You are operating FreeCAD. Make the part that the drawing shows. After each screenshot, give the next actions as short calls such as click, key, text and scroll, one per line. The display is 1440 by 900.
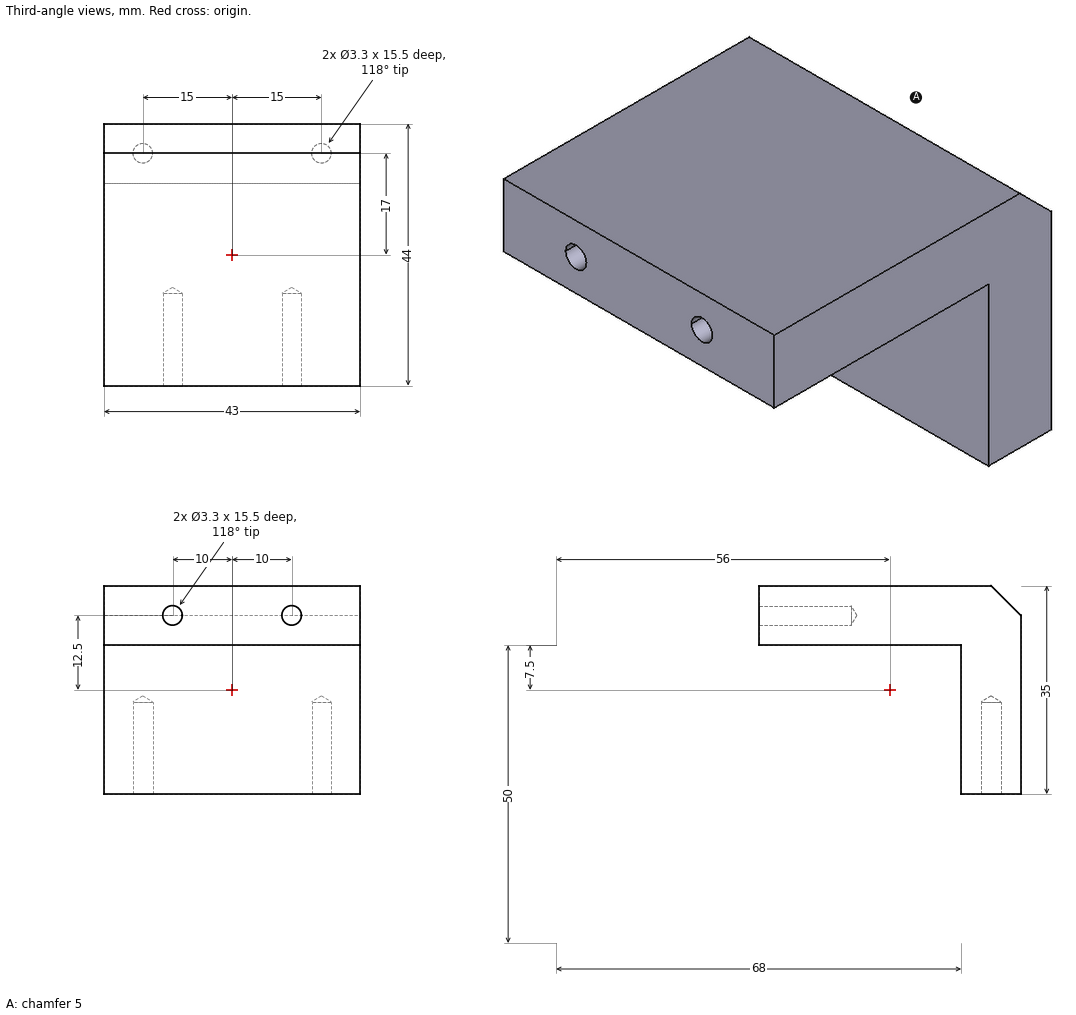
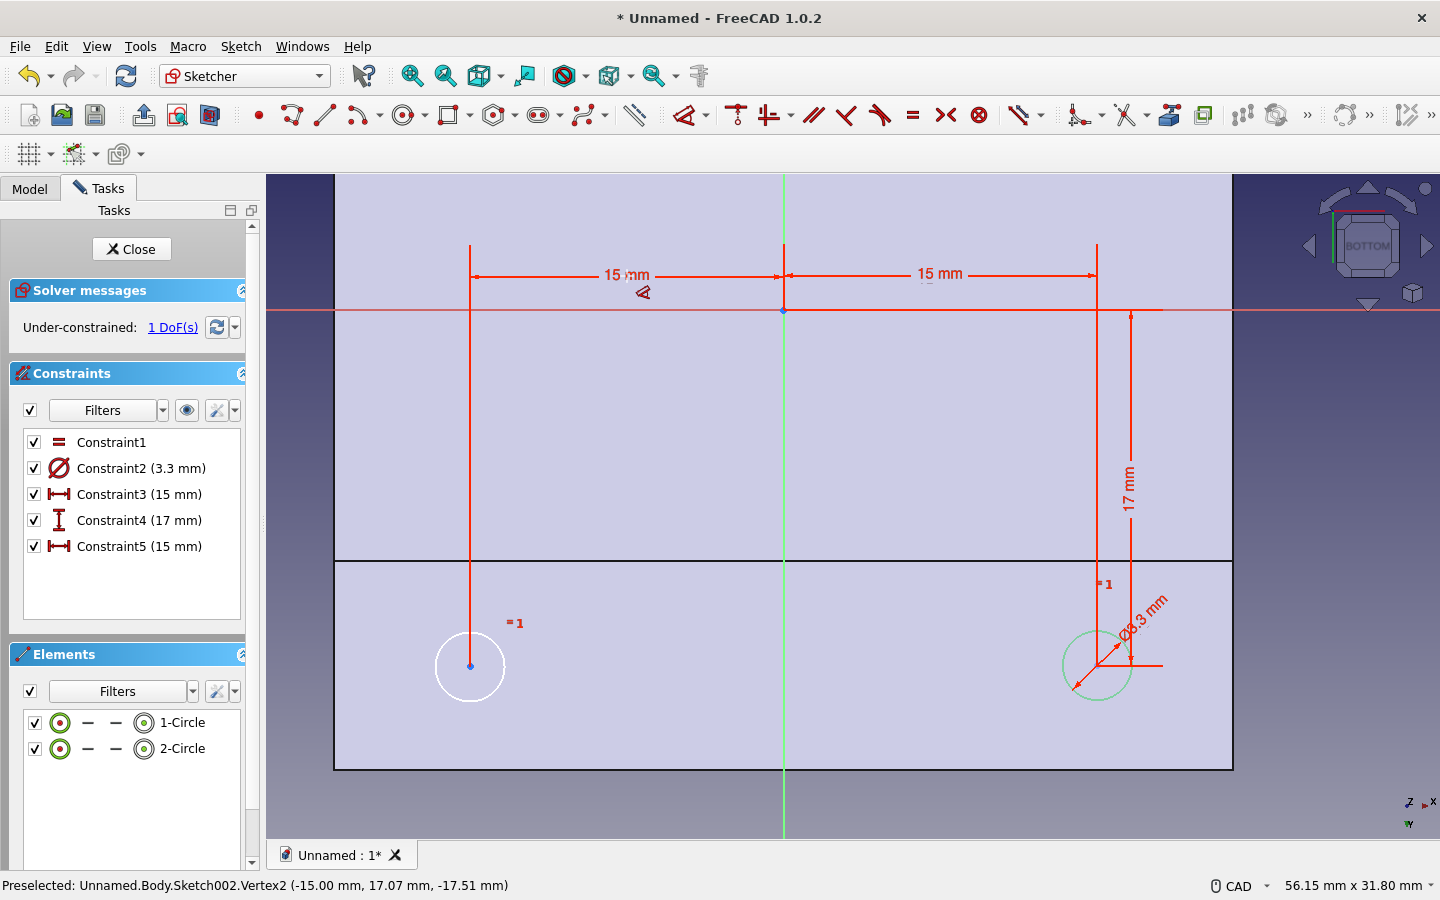
click(470, 667)
click(436, 489)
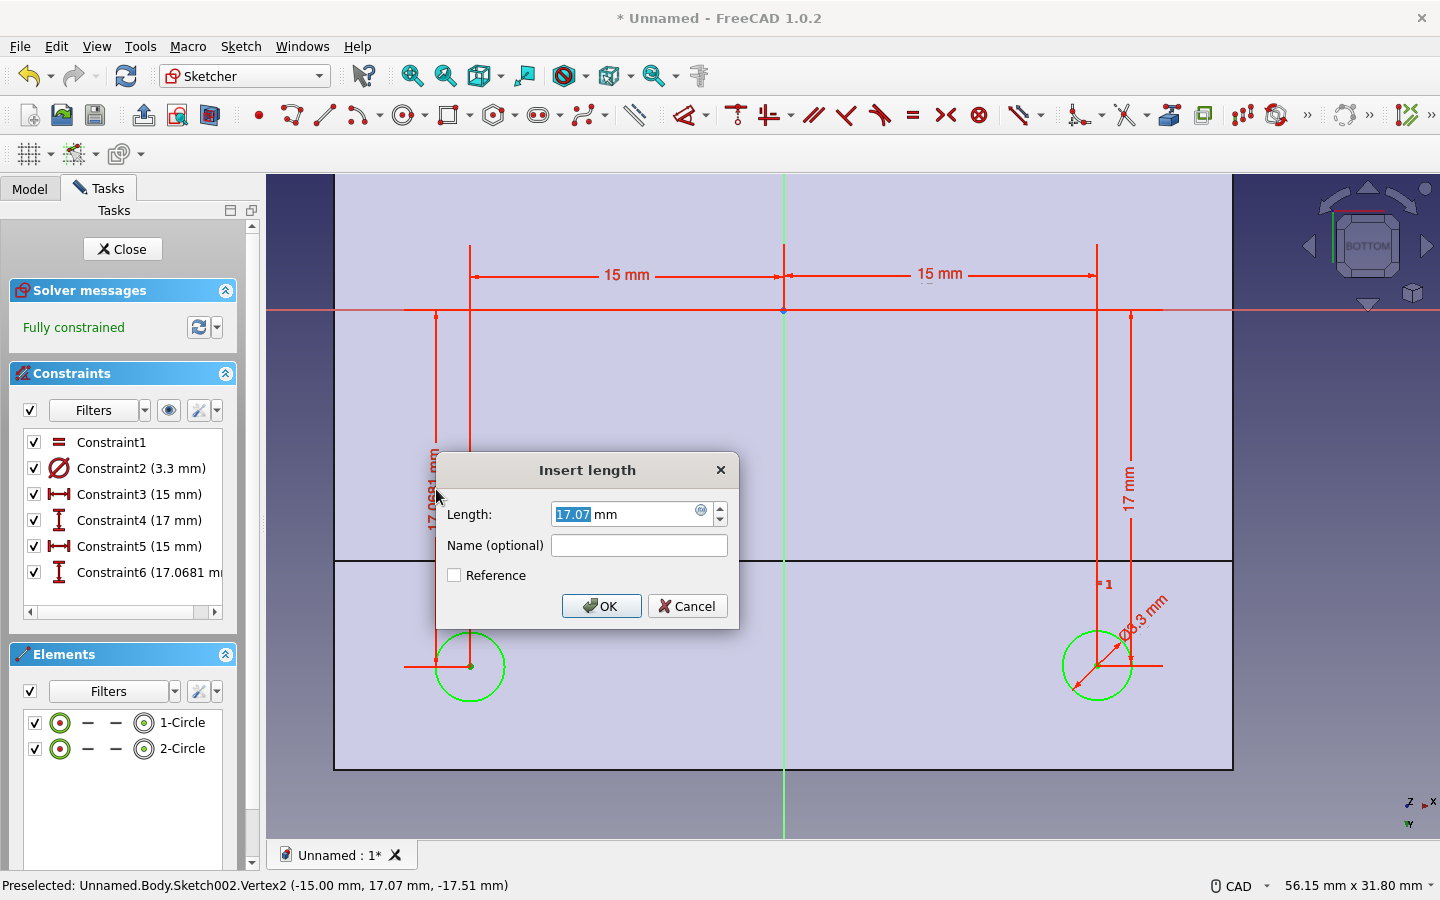
text(17)
key(Return)
key(Escape)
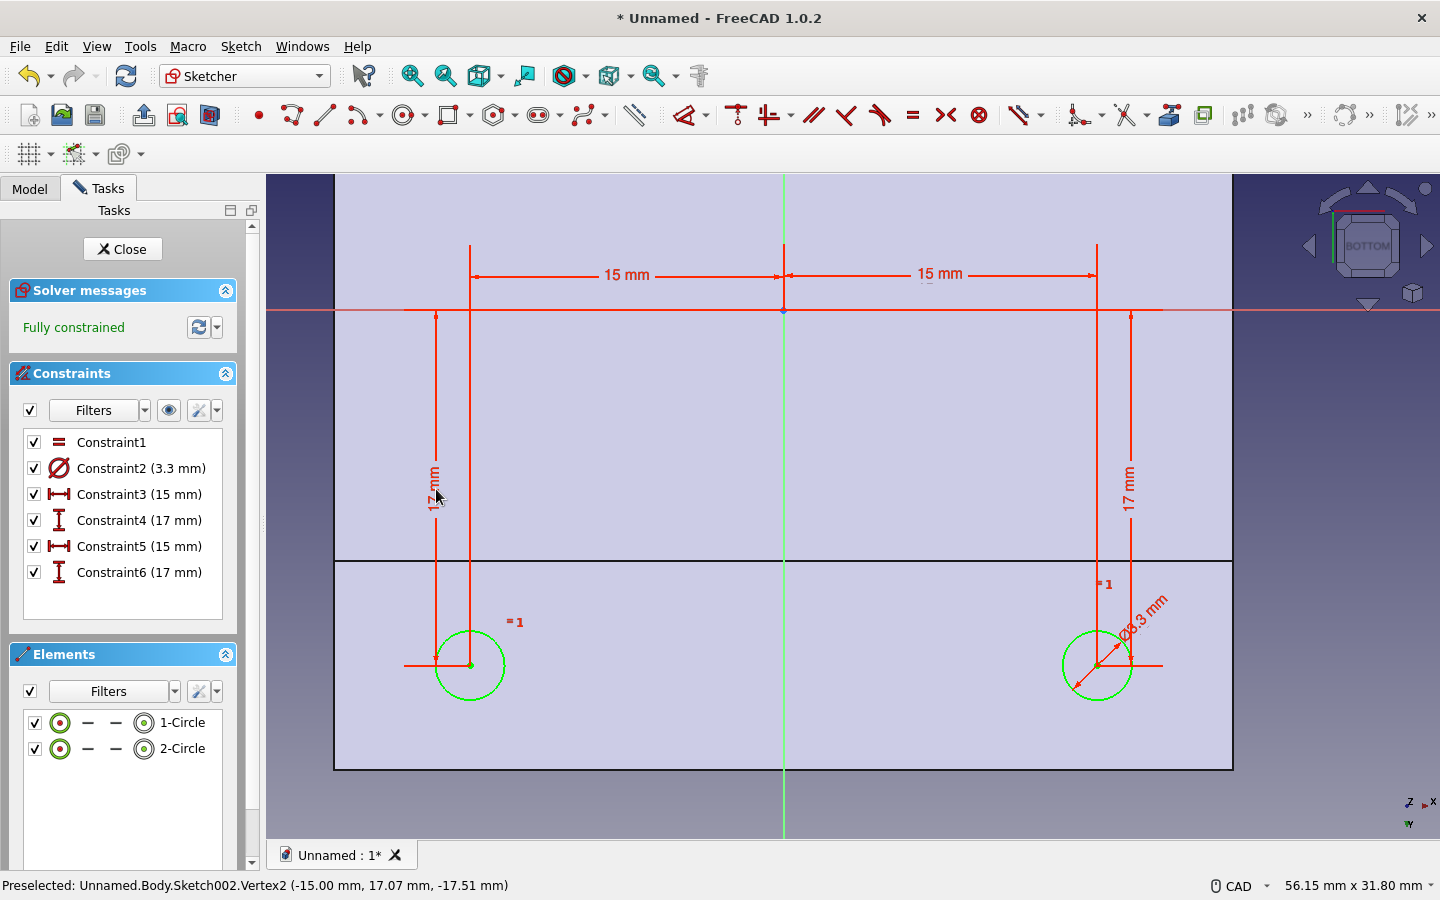
click(123, 249)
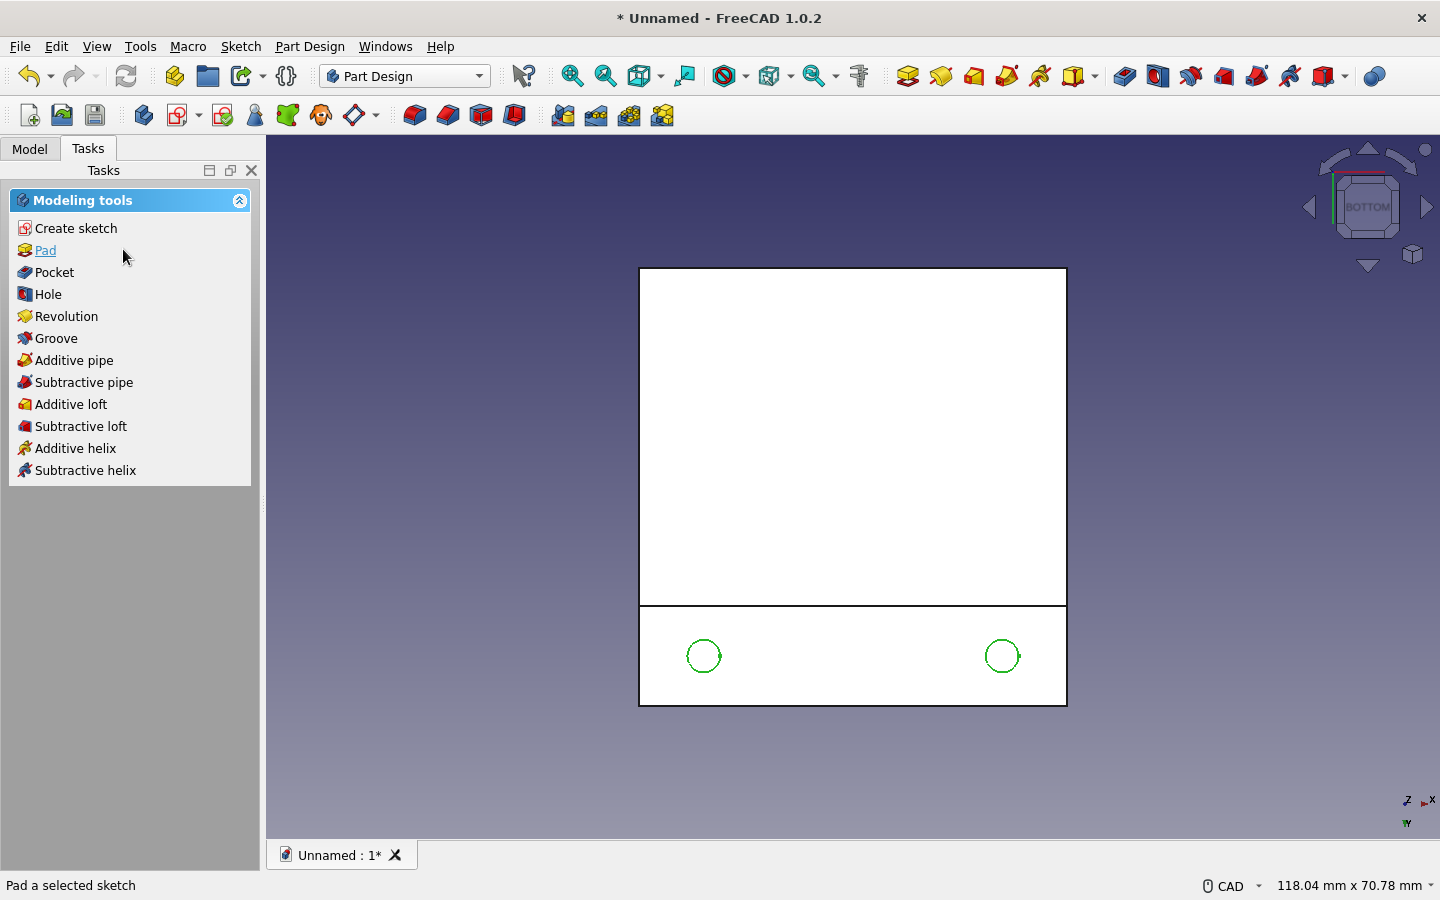
click(1158, 76)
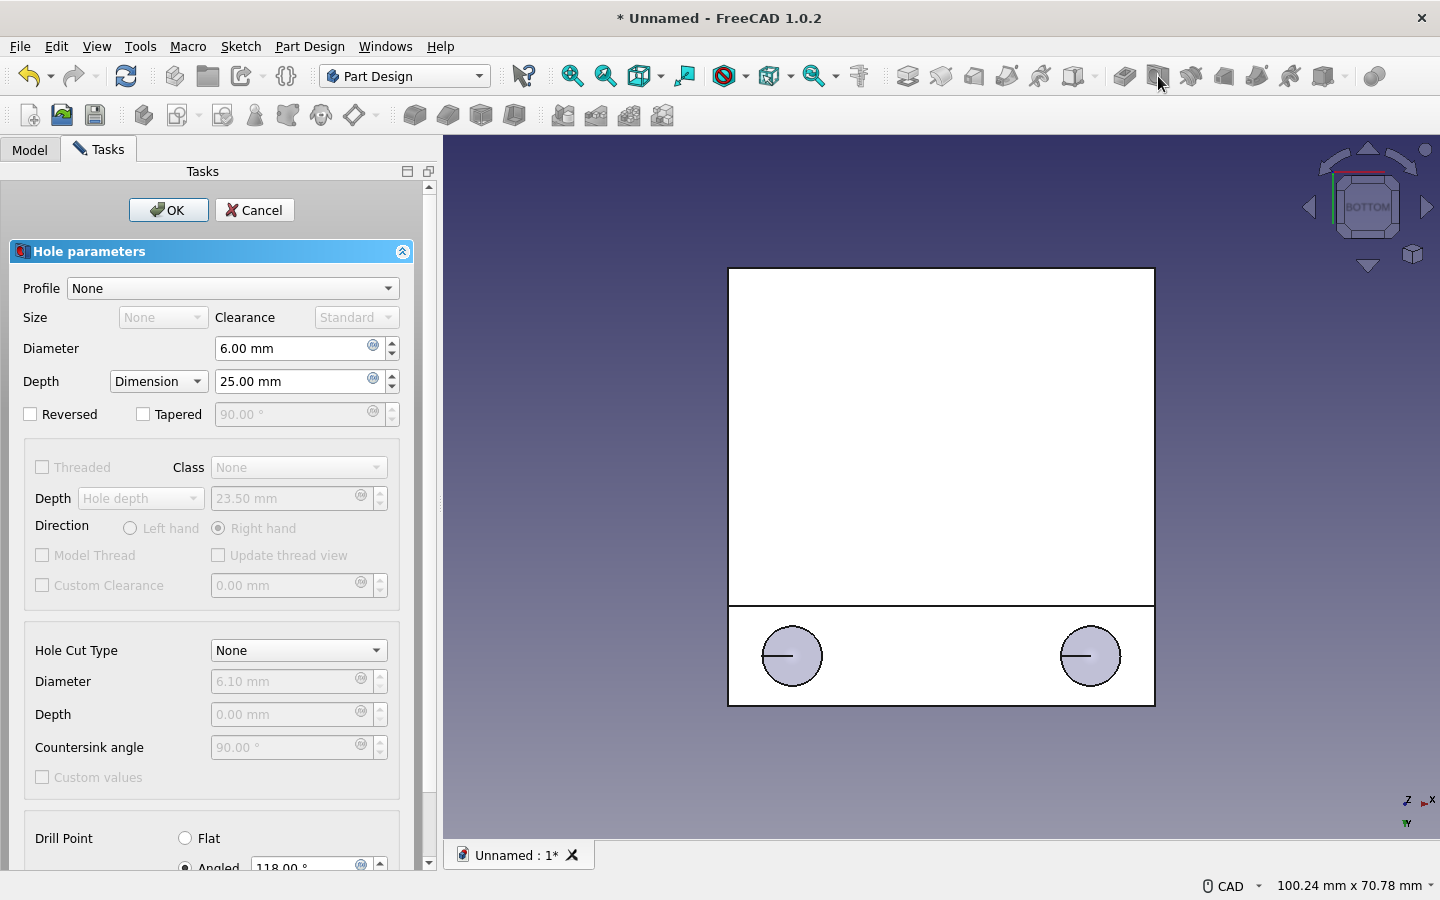
triple_click(300, 348)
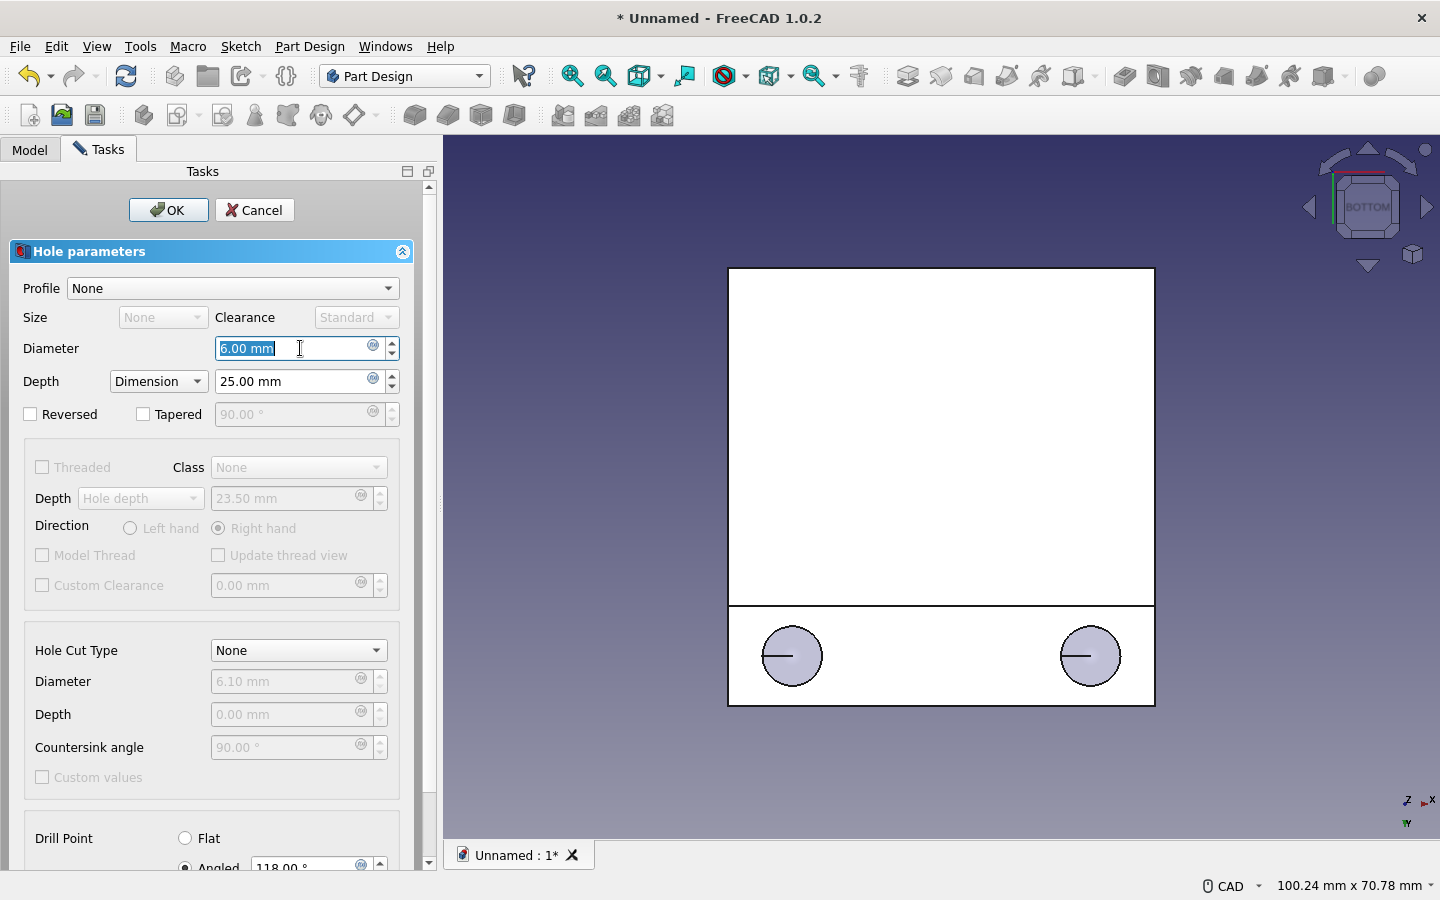
text(3.3)
key(Tab)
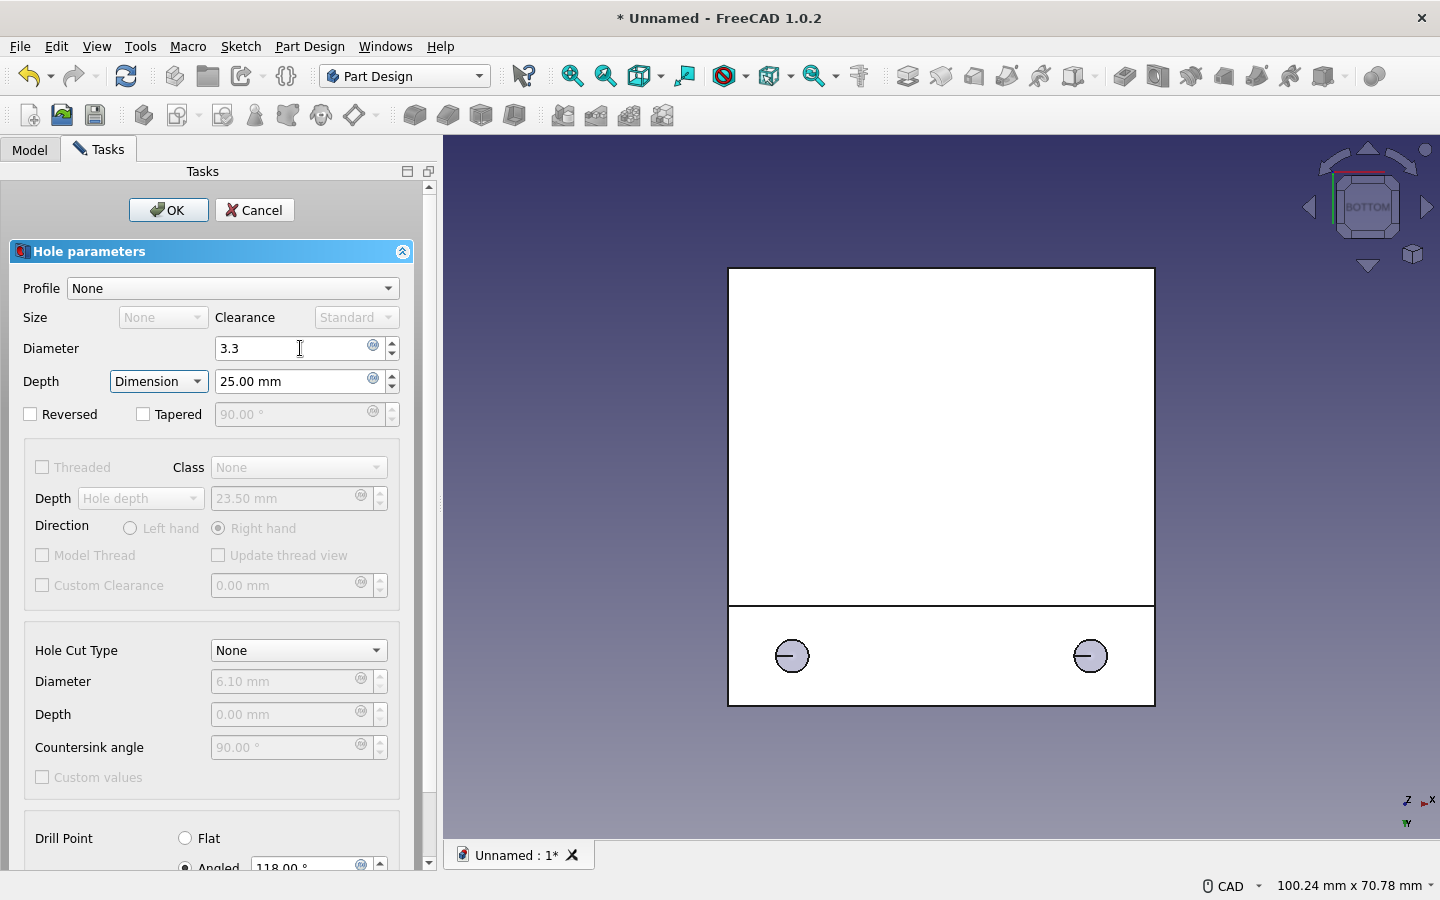
triple_click(300, 382)